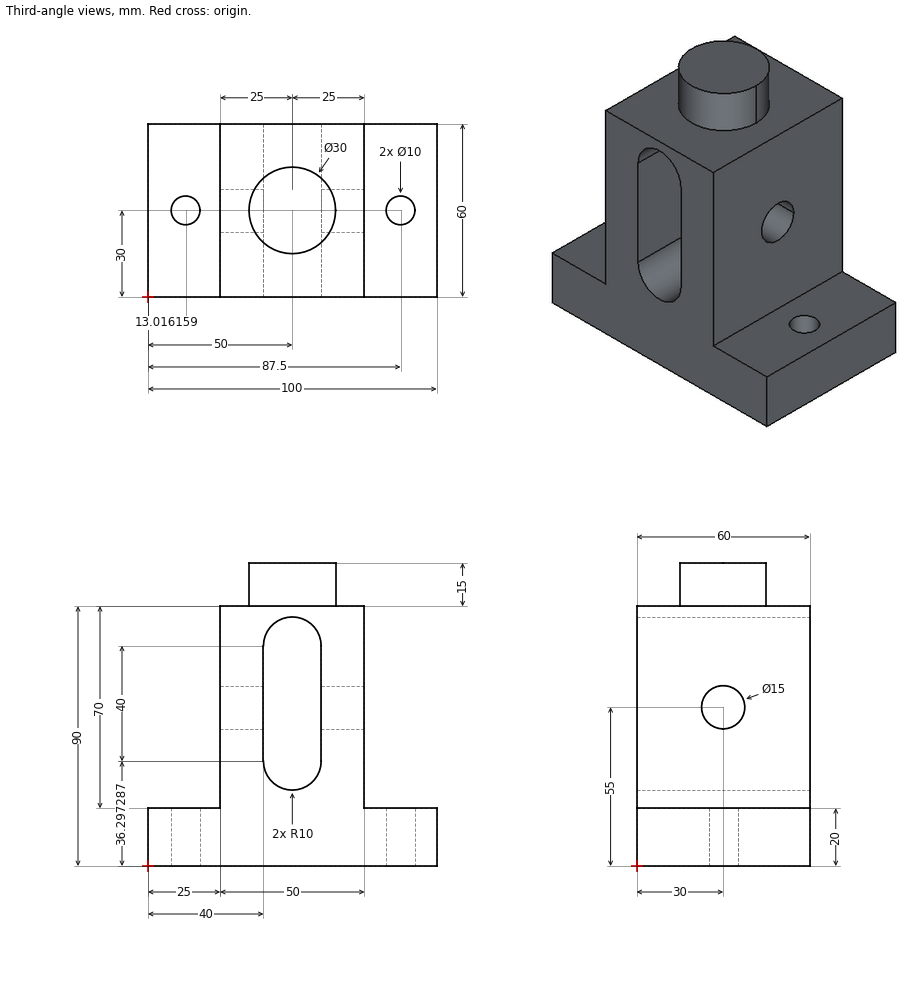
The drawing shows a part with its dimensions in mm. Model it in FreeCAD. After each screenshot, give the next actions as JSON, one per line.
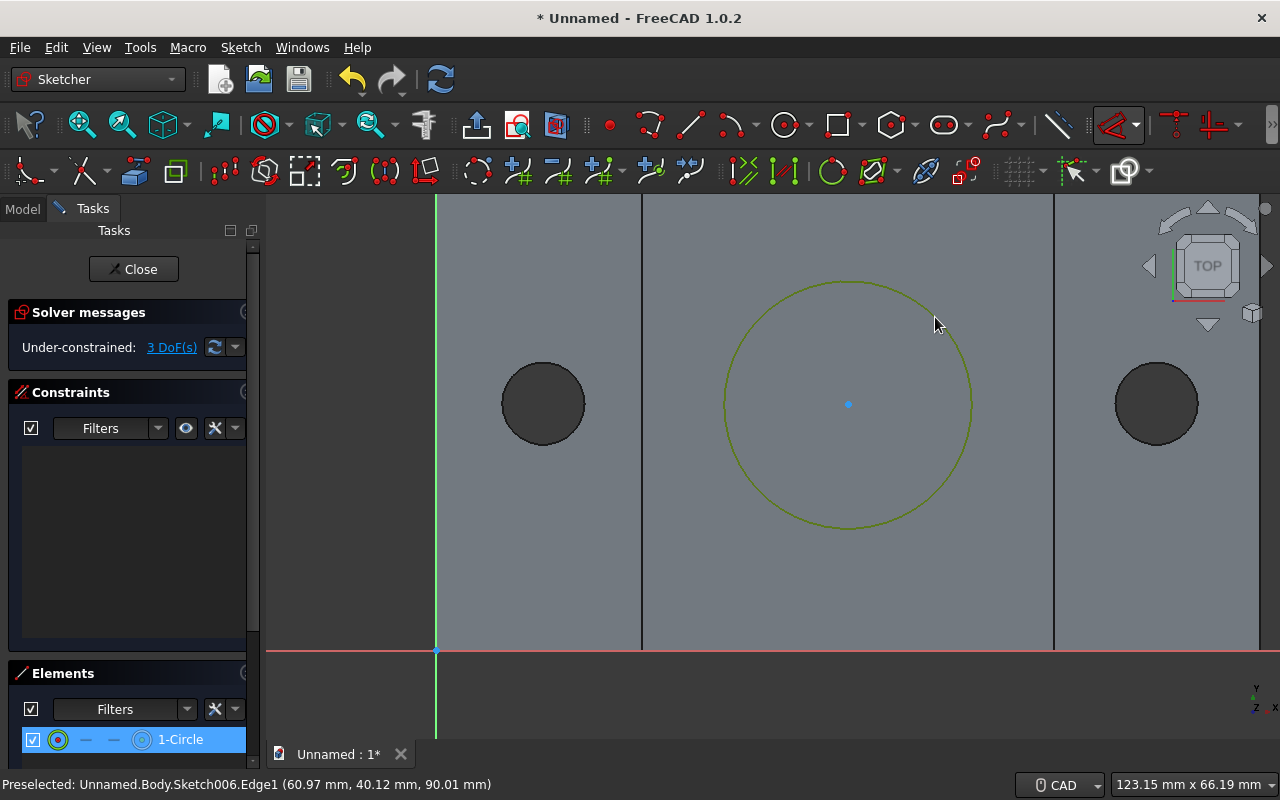
{"action": "left_click", "coordinate": [1138, 126]}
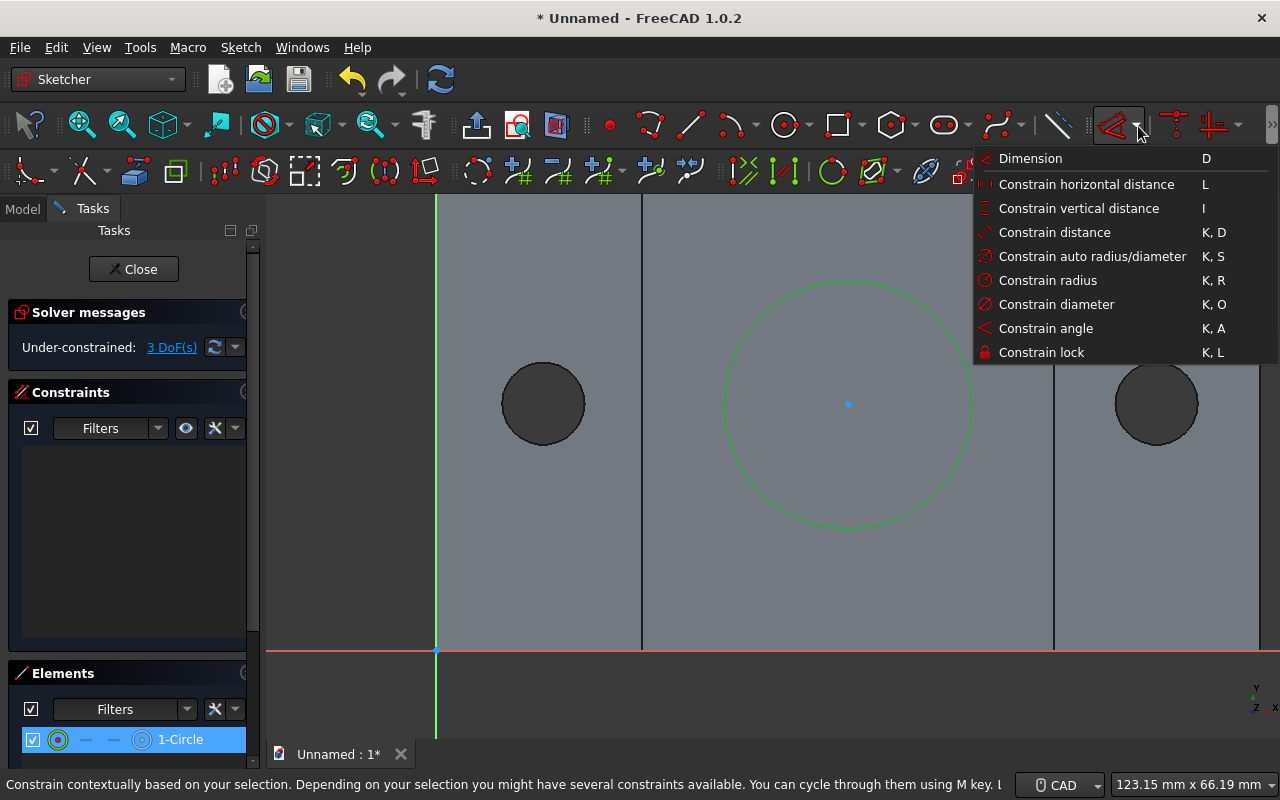
{"action": "left_click", "coordinate": [1126, 304]}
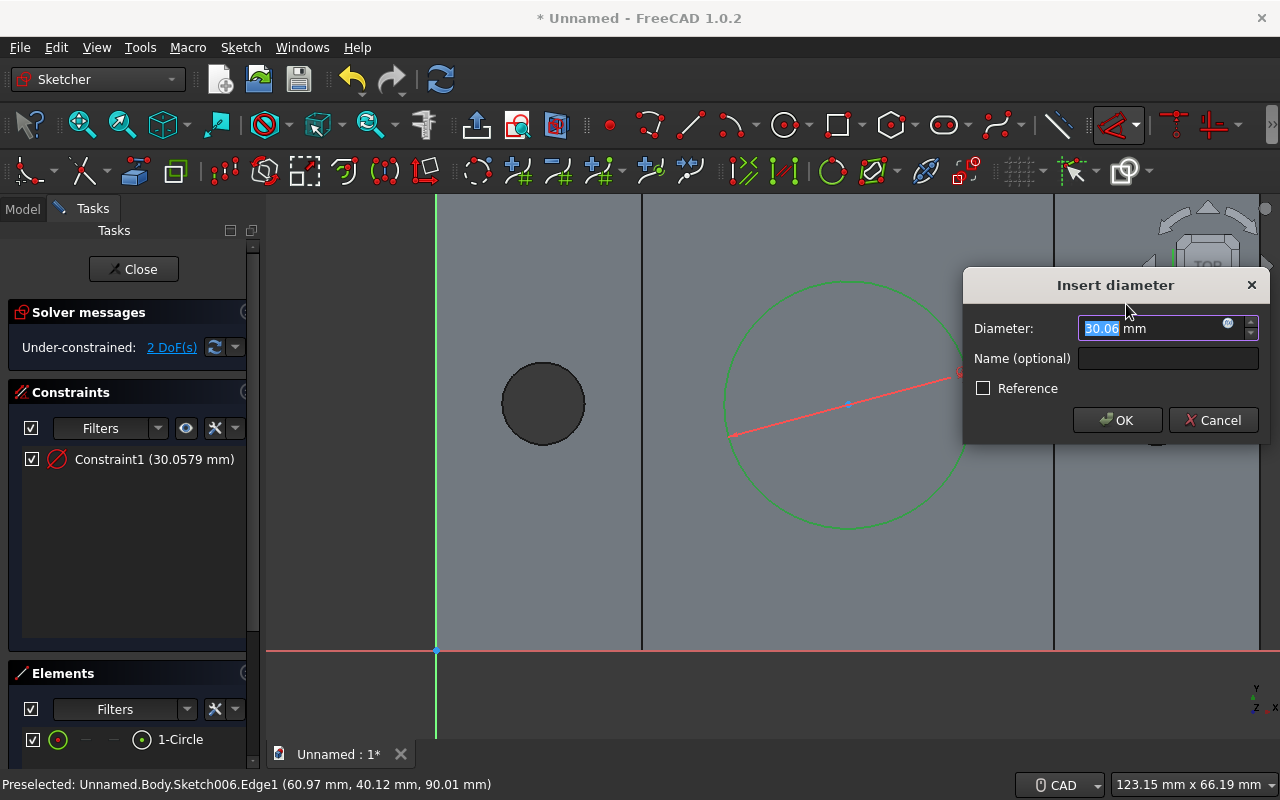
{"action": "type", "text": "30"}
{"action": "key", "text": "Return"}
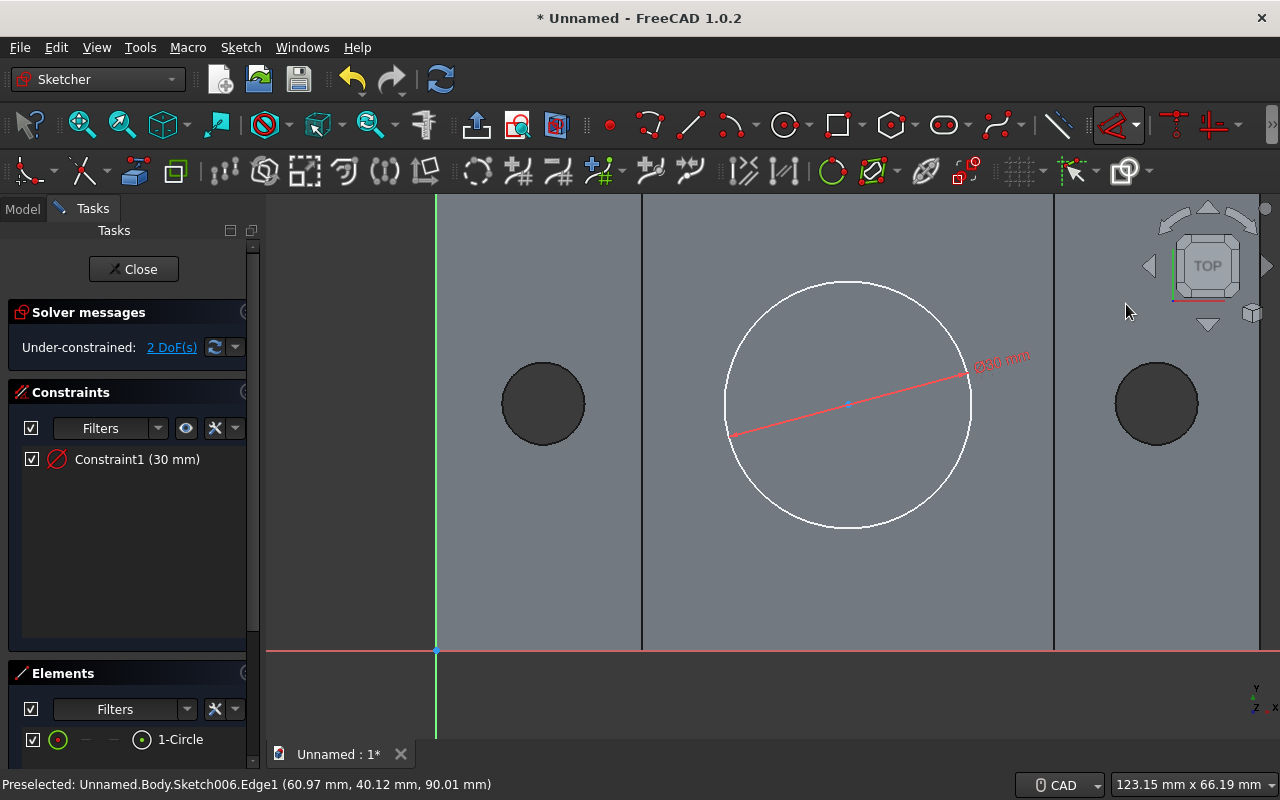
{"action": "left_click", "coordinate": [848, 405]}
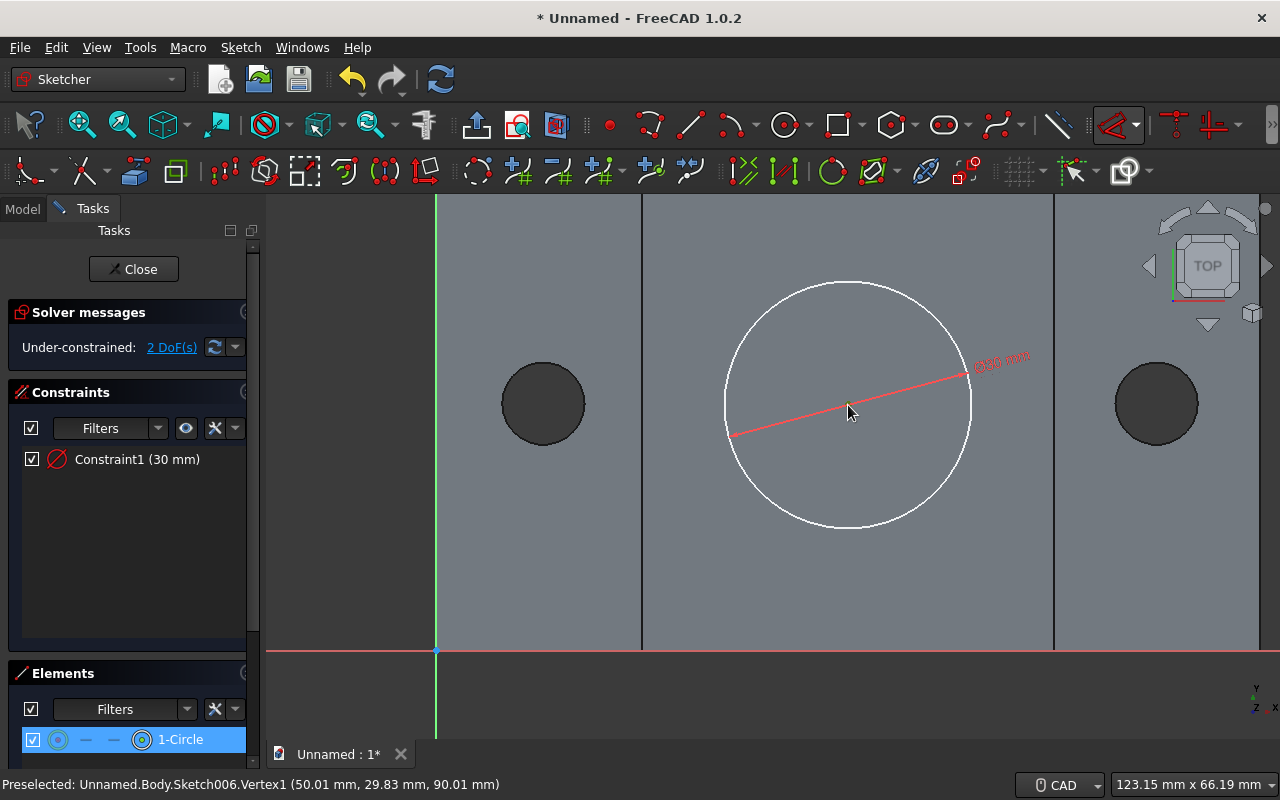
{"action": "key", "text": "l"}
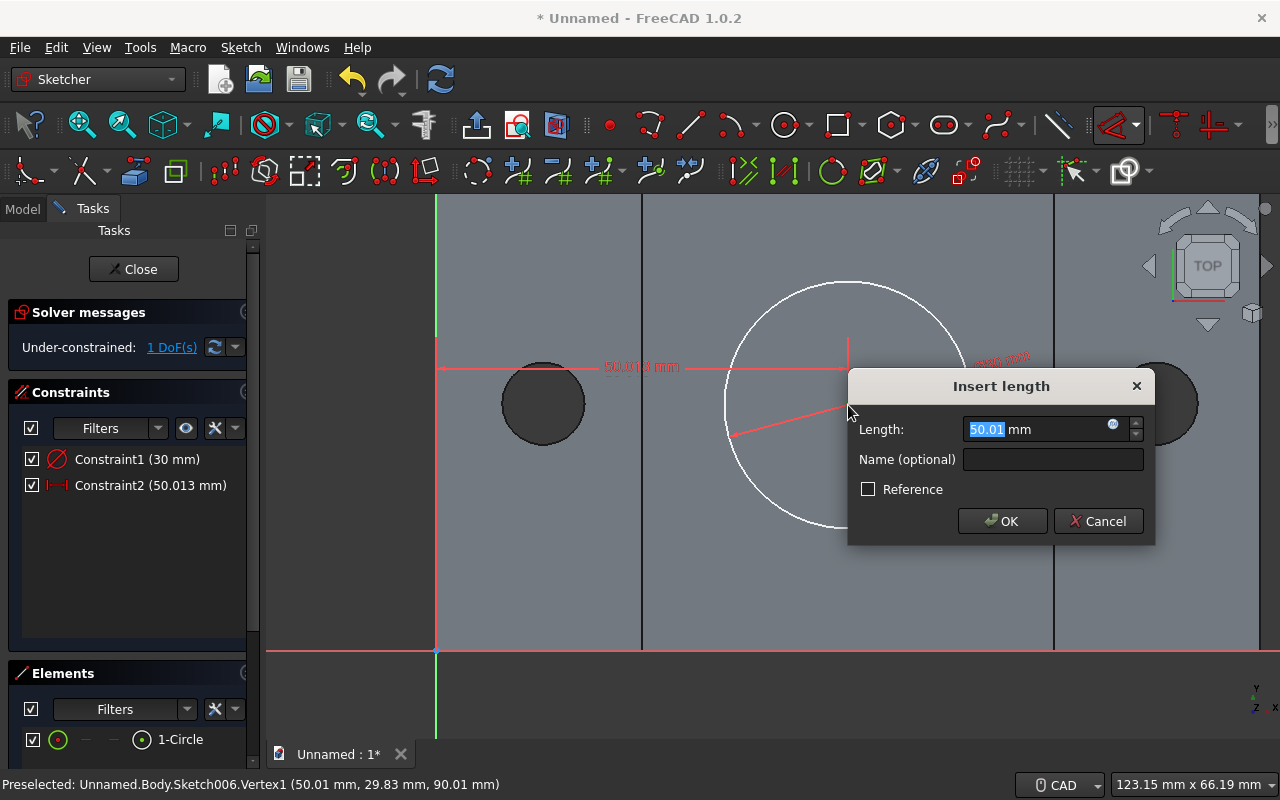
{"action": "type", "text": "50"}
{"action": "key", "text": "Return"}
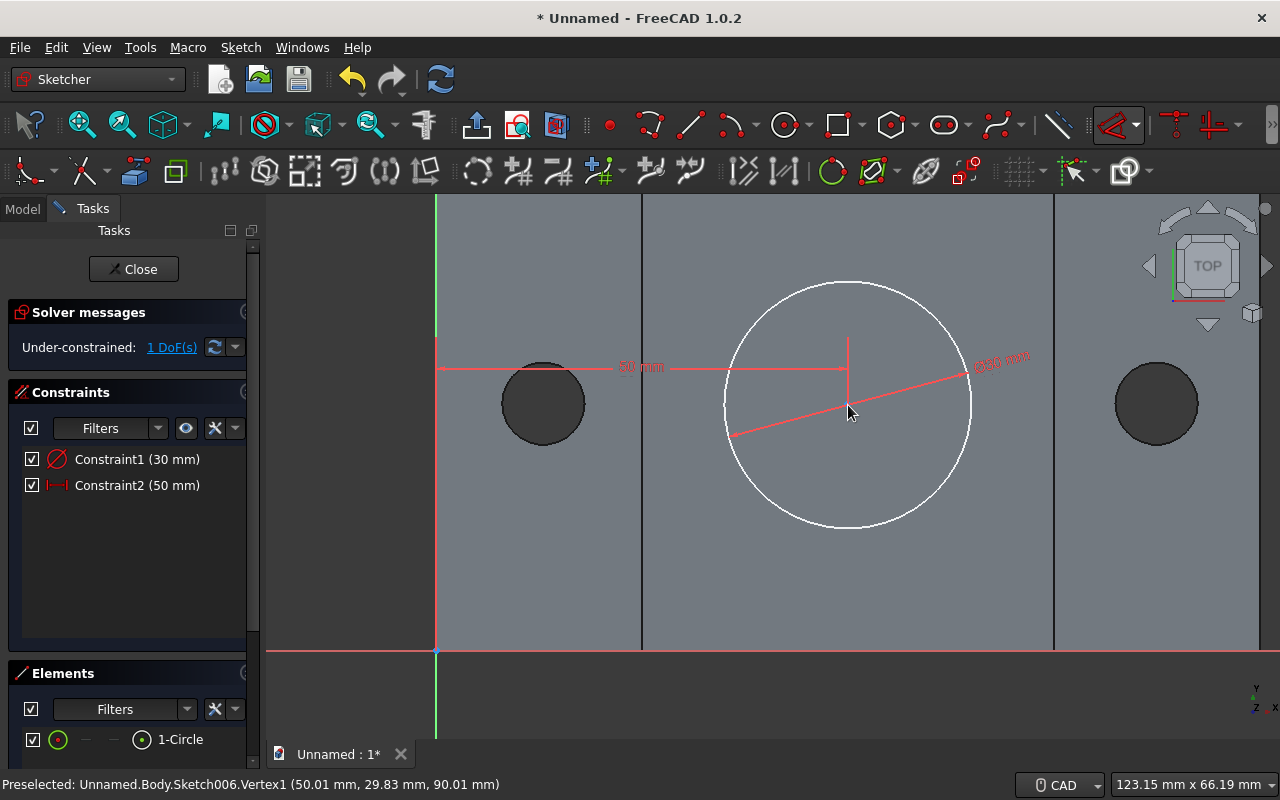
{"action": "left_click", "coordinate": [848, 405]}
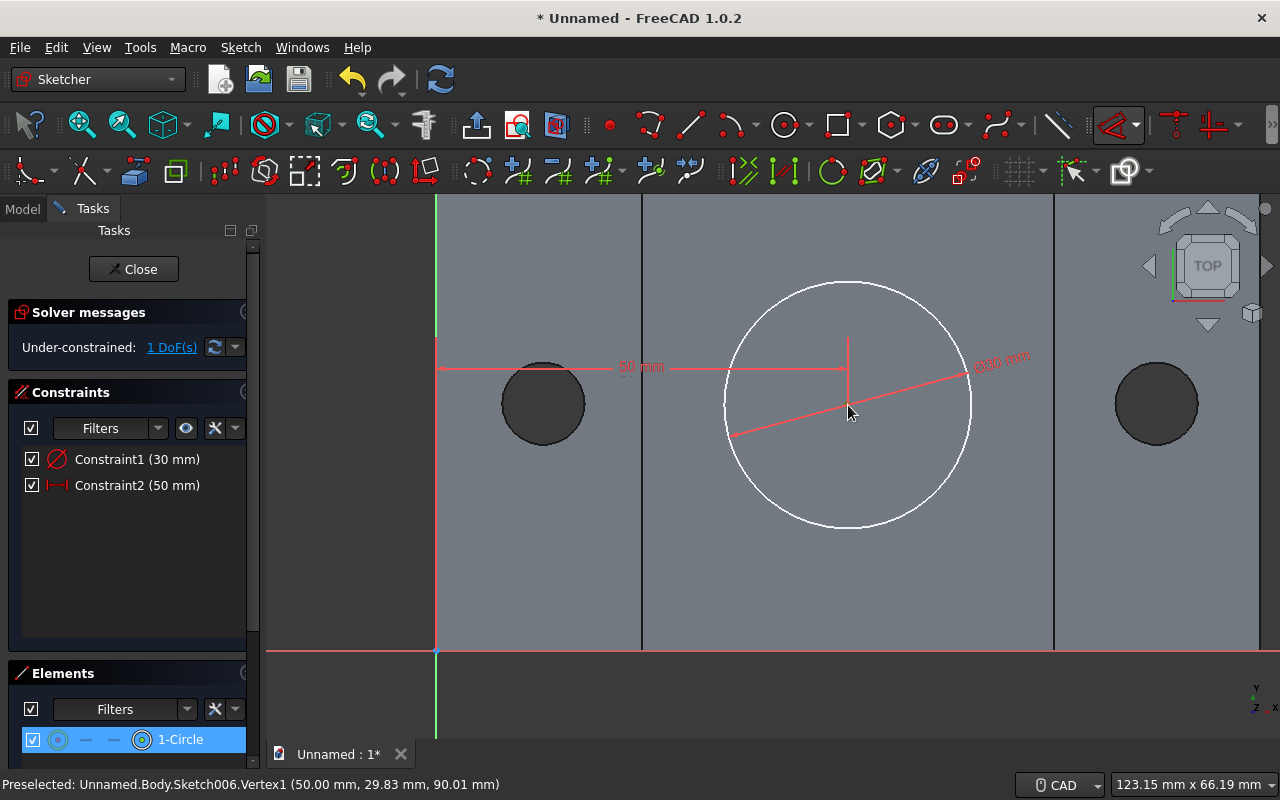
{"action": "left_click", "coordinate": [1138, 126]}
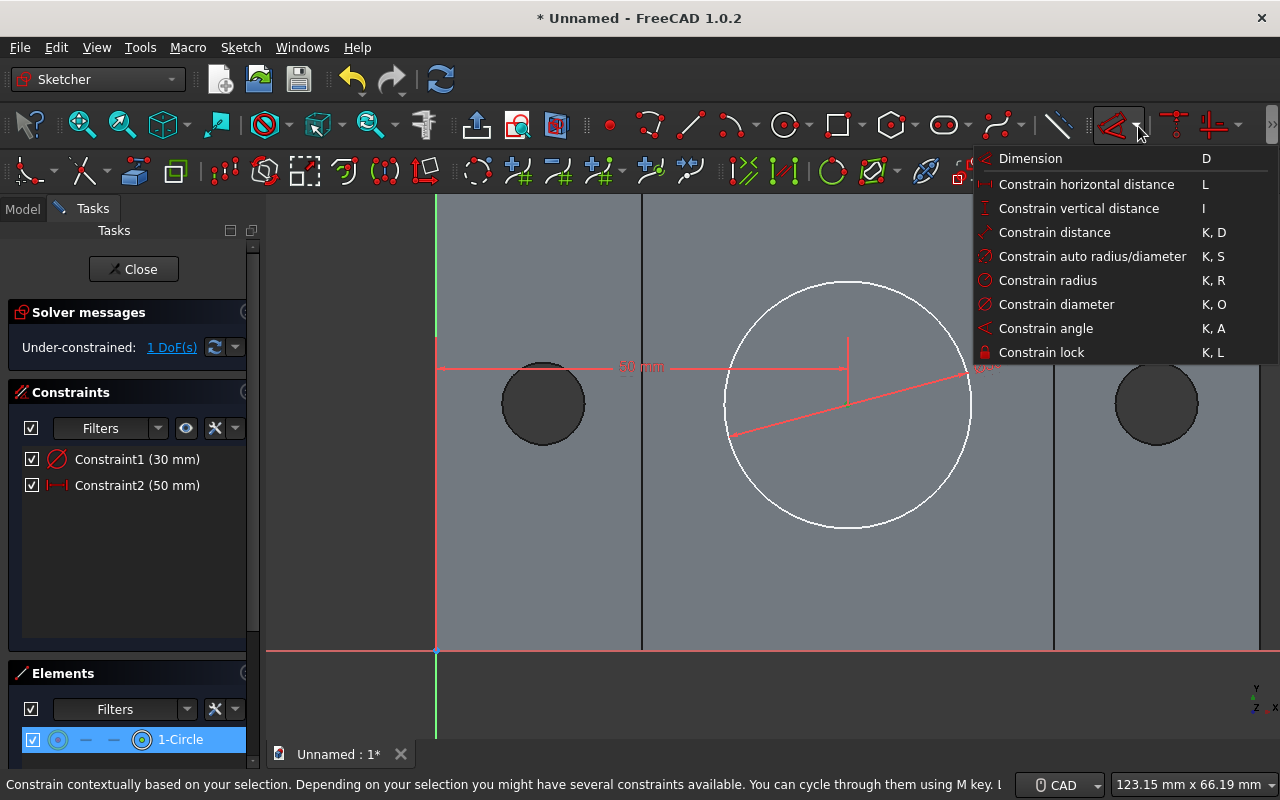
{"action": "left_click", "coordinate": [1126, 208]}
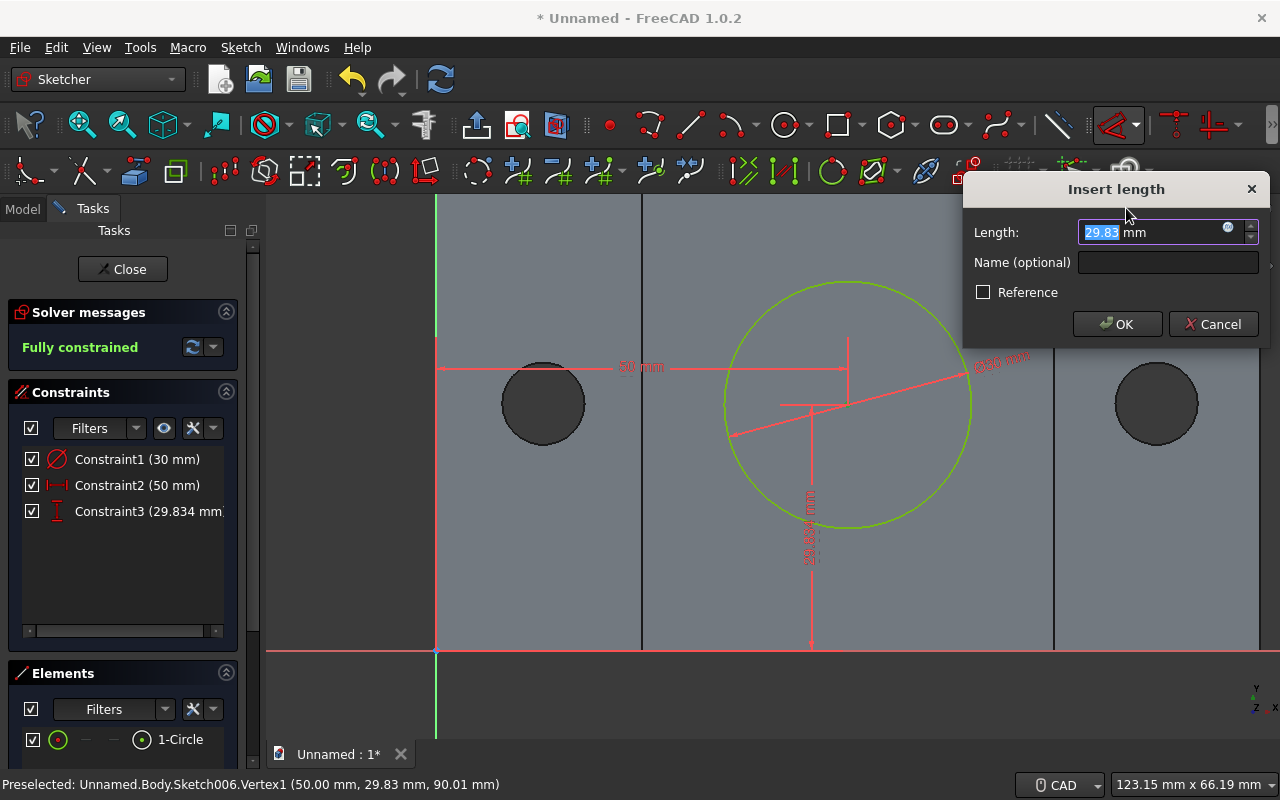
{"action": "type", "text": "30"}
{"action": "key", "text": "Return"}